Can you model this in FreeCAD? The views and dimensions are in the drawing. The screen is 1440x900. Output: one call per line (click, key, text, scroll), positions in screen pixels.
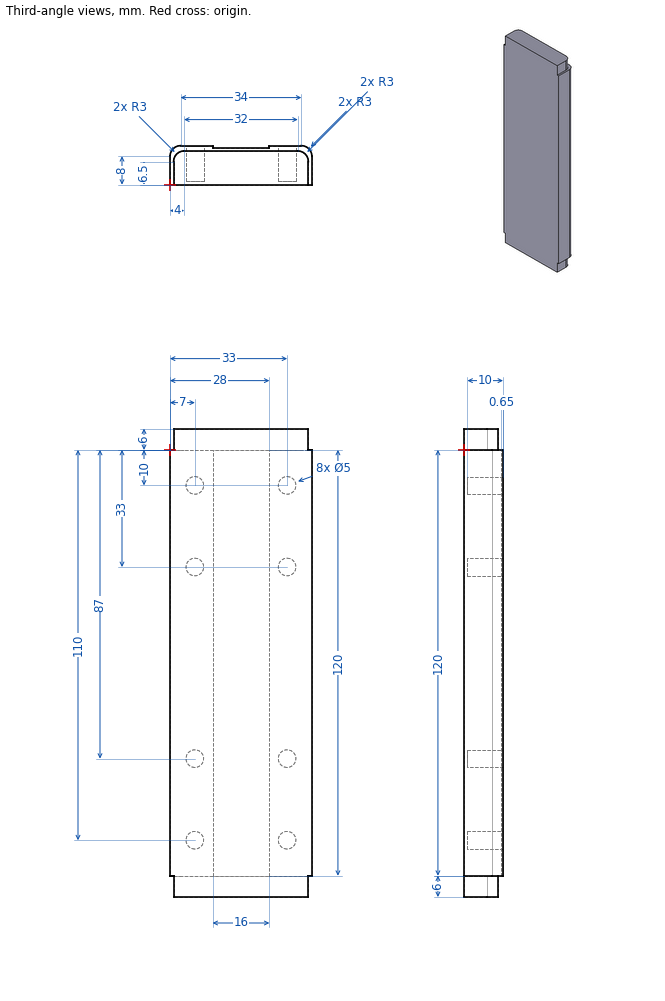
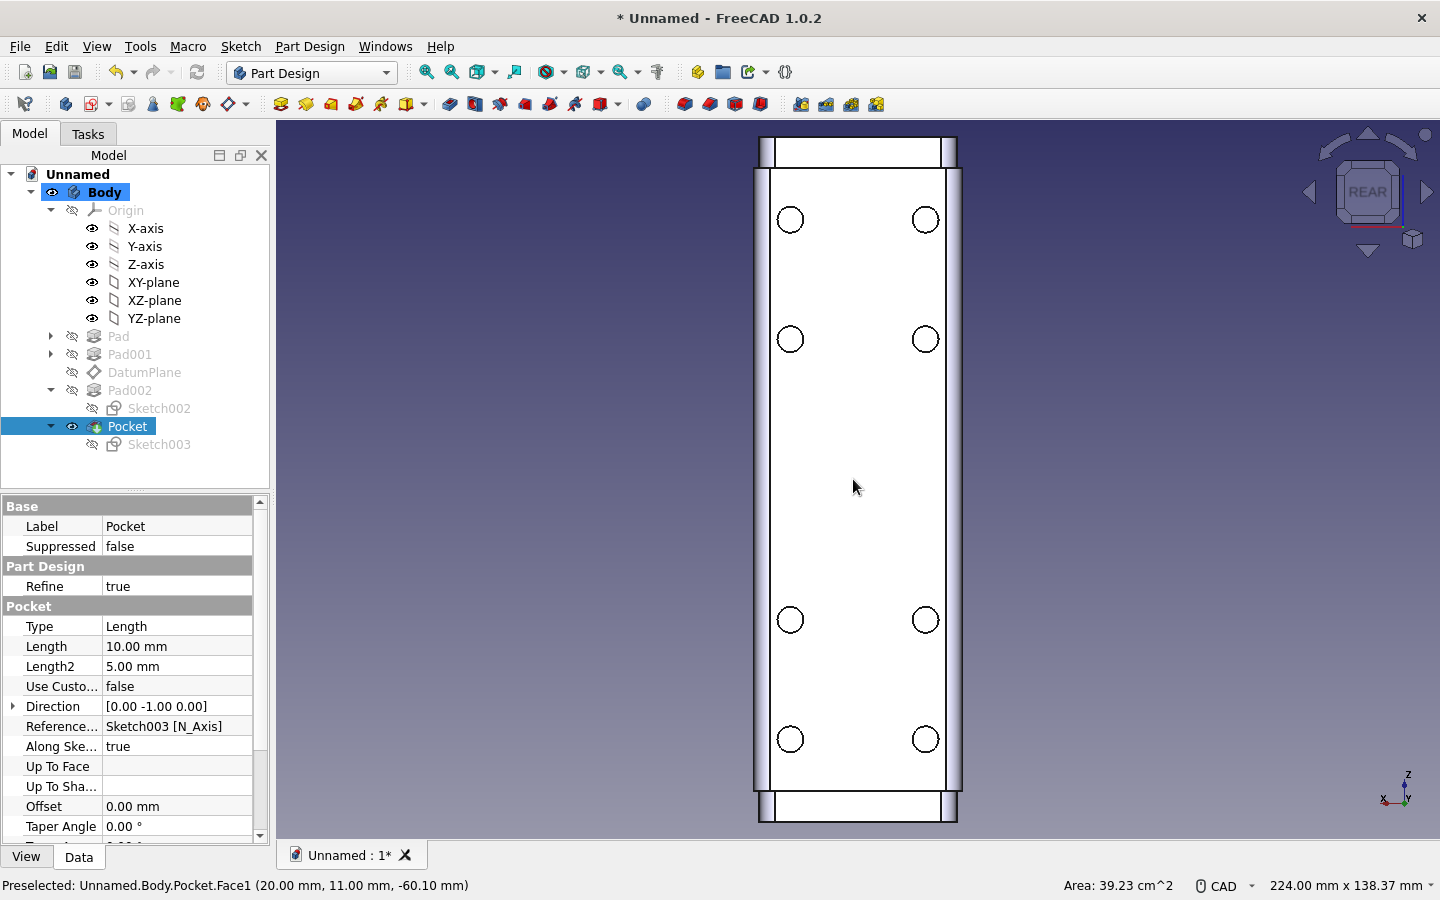
click(90, 104)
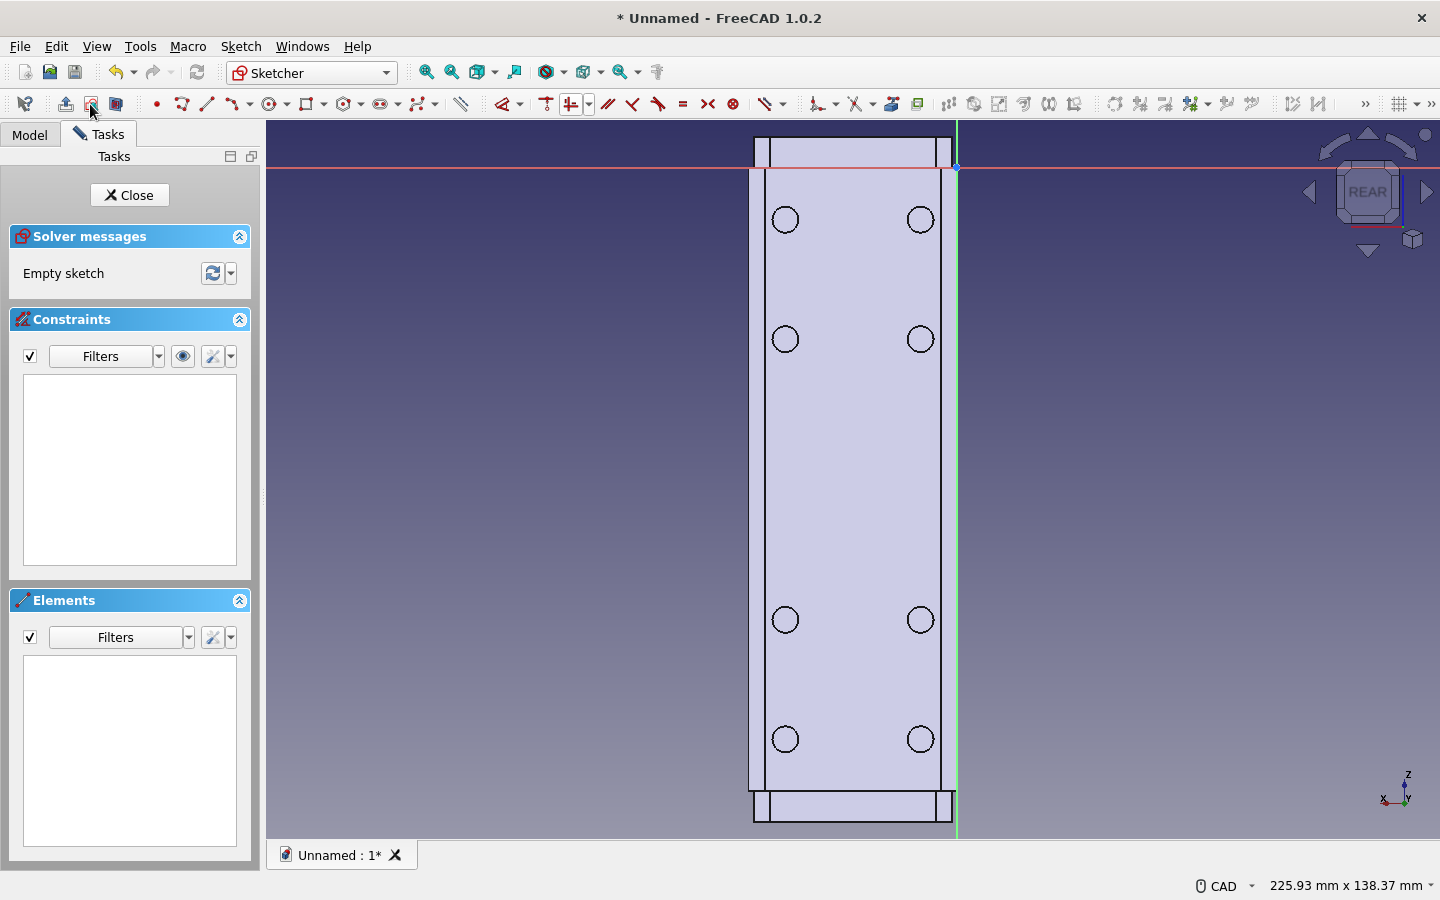
scroll(334, 479, down, 1)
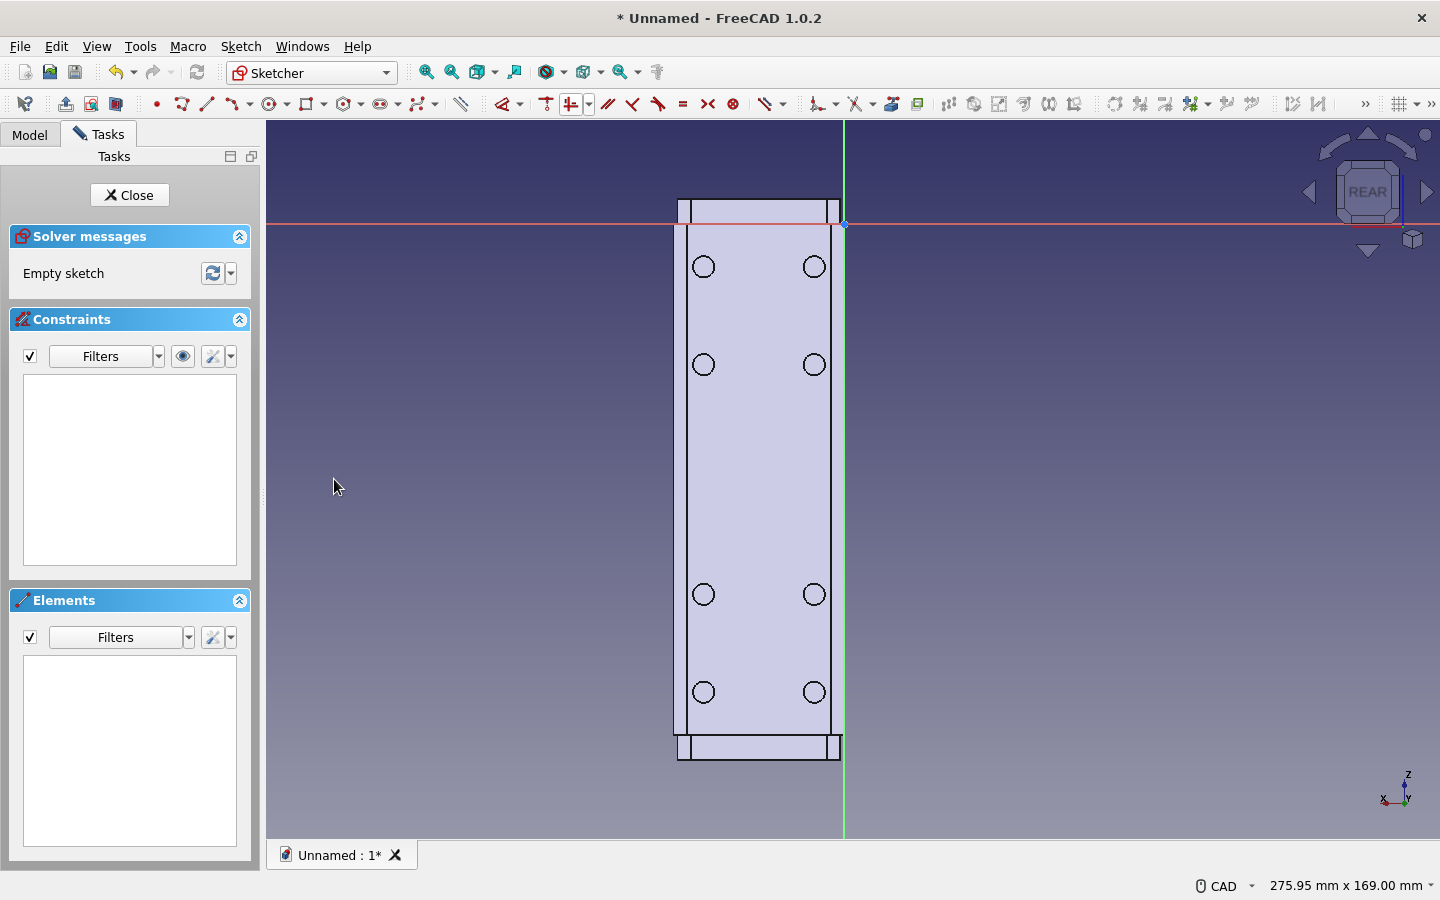
click(306, 104)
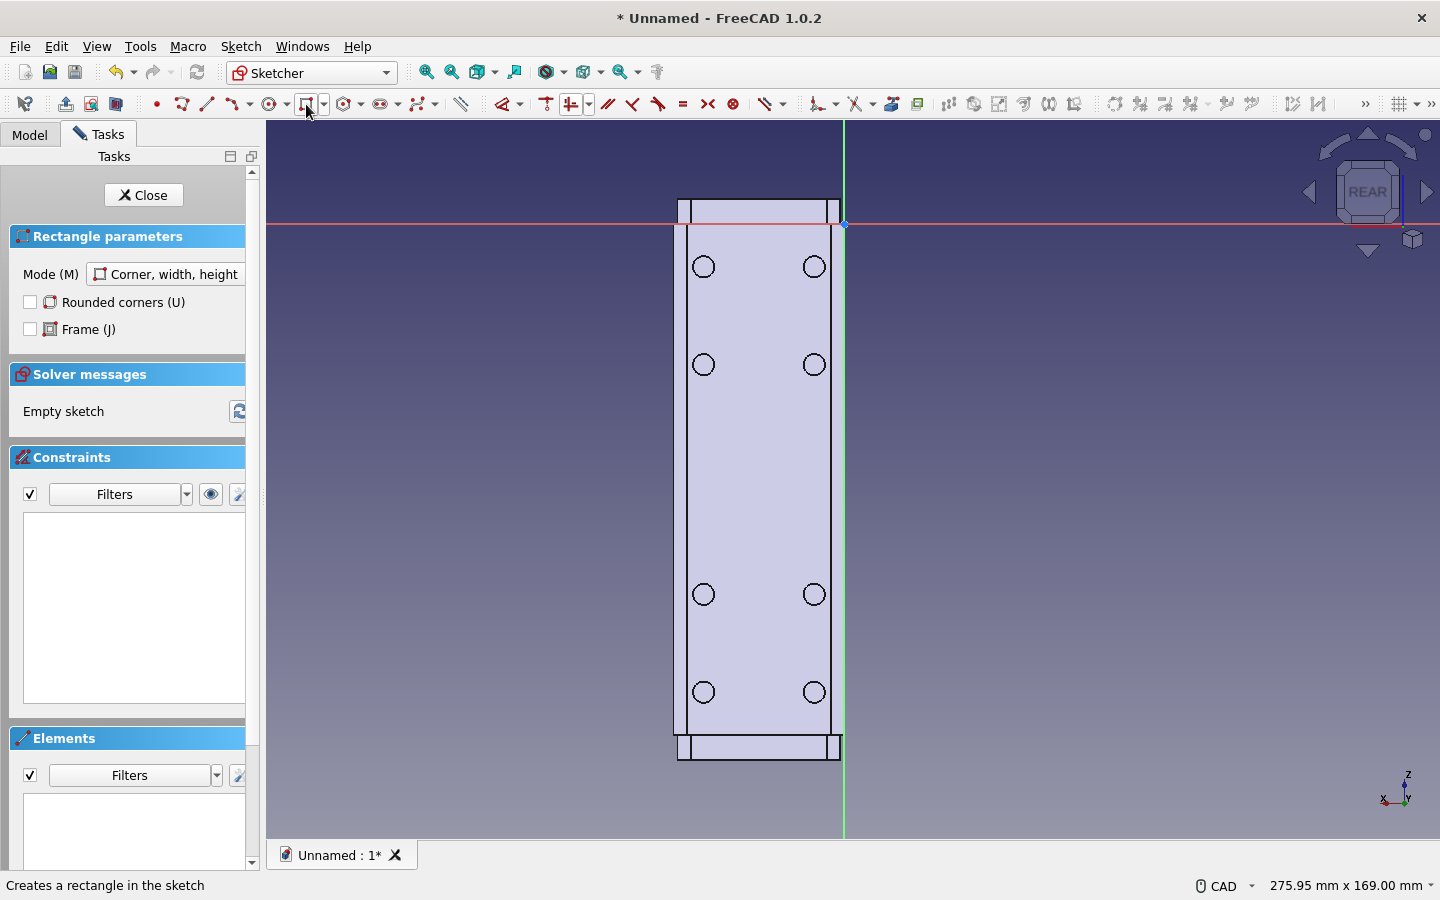
click(725, 224)
click(793, 735)
key(Escape)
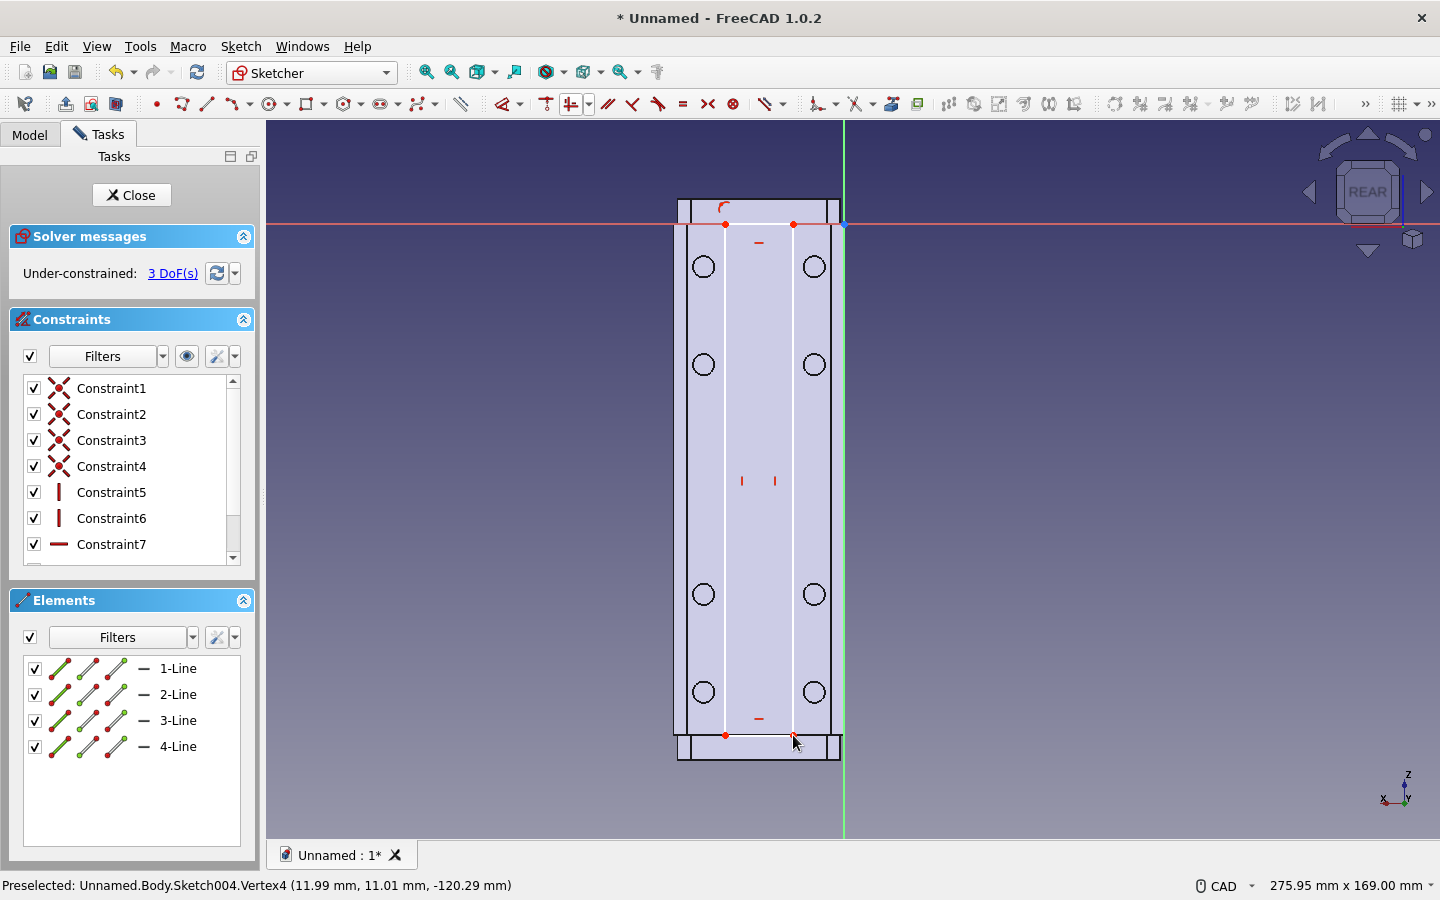
click(502, 104)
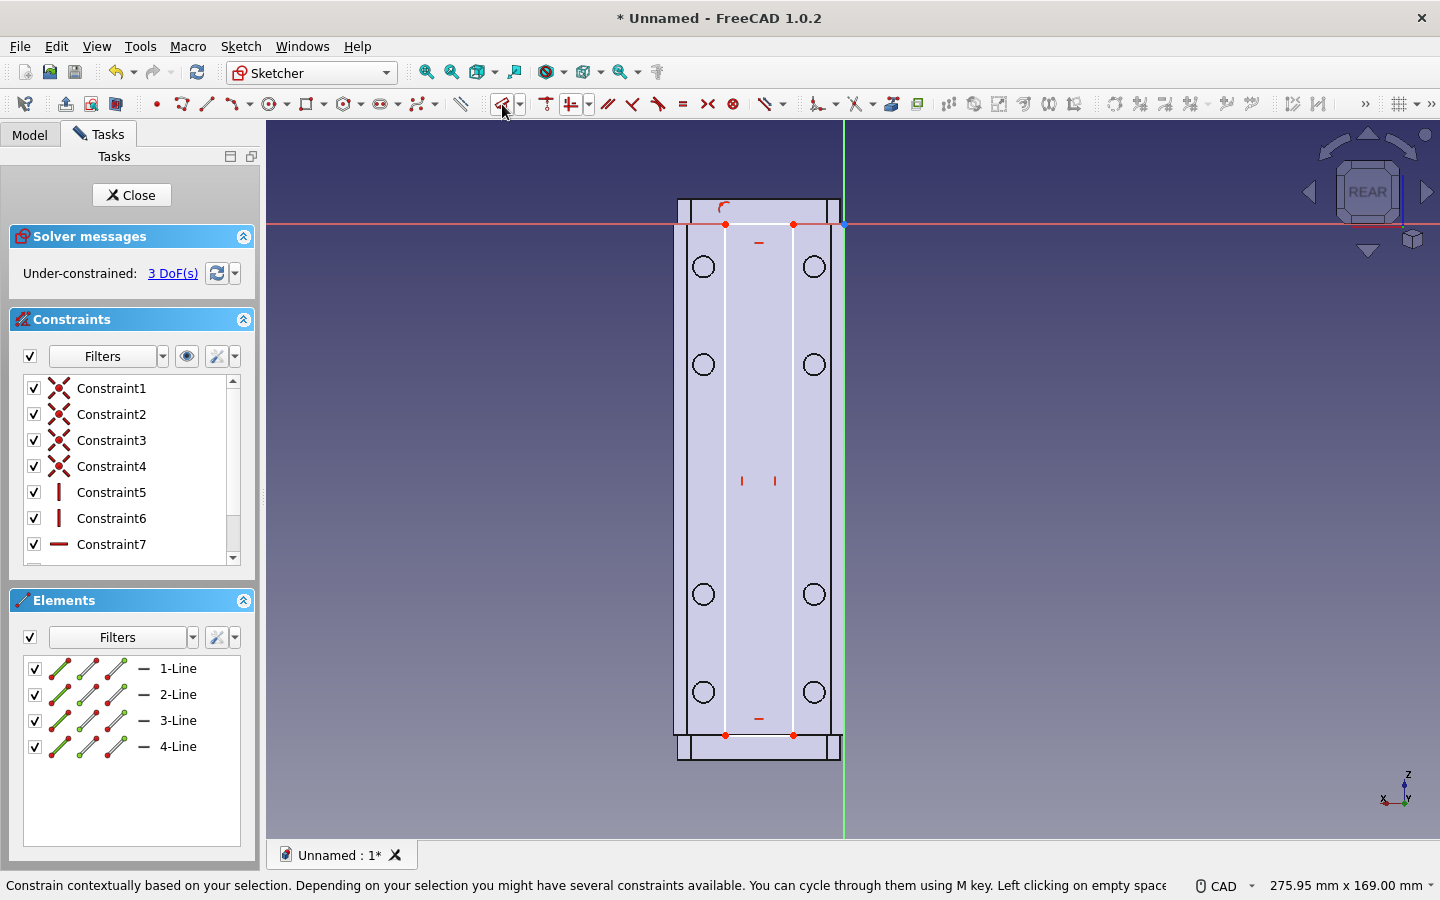
click(745, 736)
click(759, 770)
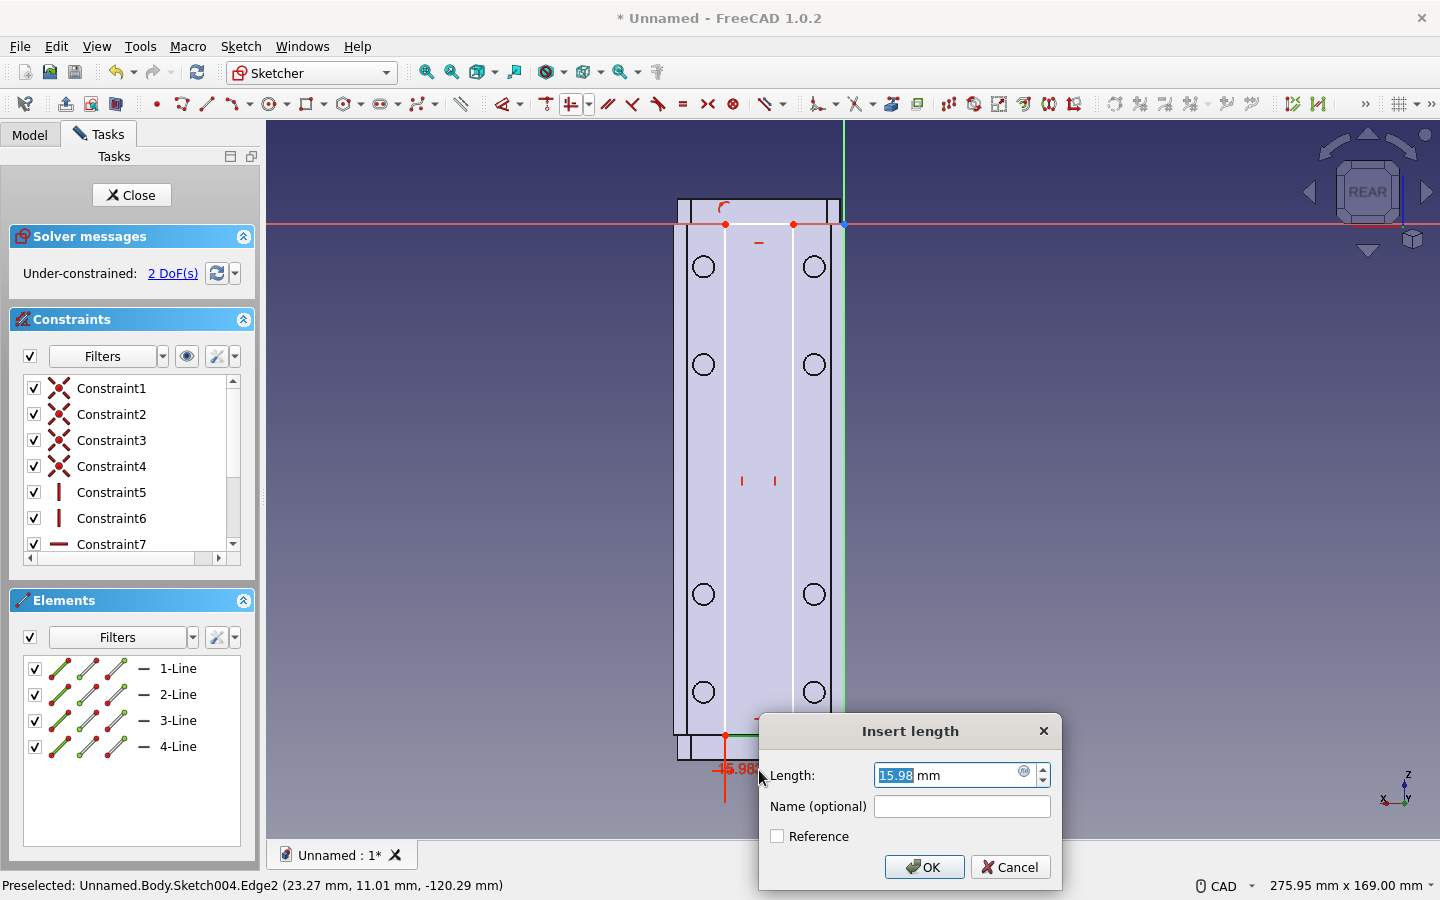
text(16)
key(Return)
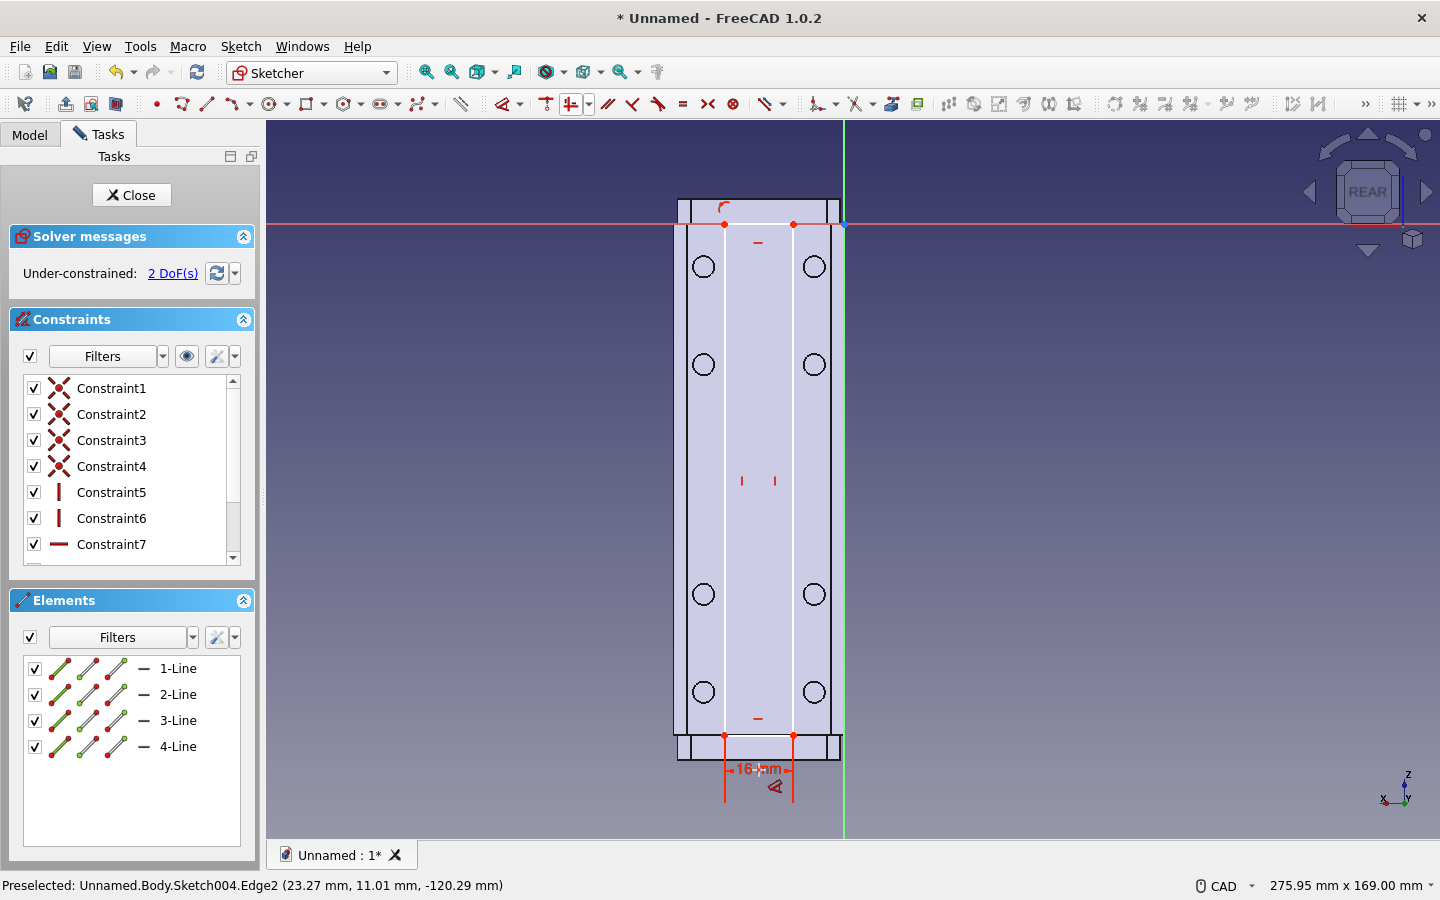
click(725, 378)
click(691, 480)